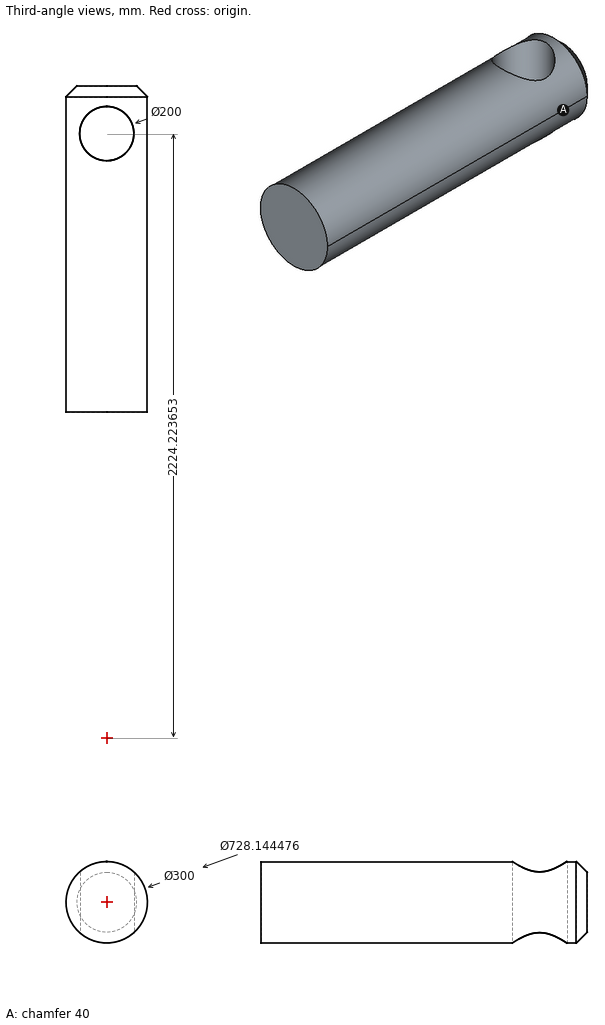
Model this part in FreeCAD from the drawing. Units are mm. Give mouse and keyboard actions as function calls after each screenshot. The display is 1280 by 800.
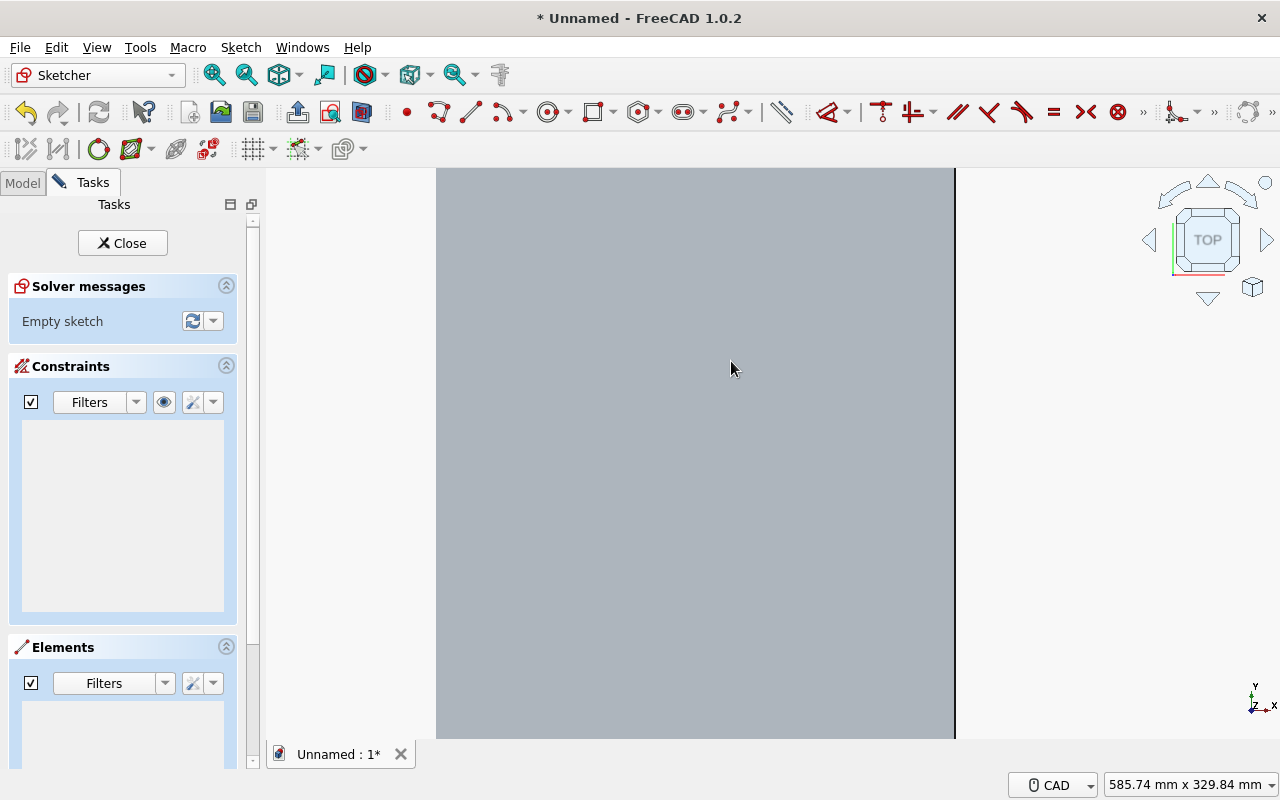
key(g)
key(c)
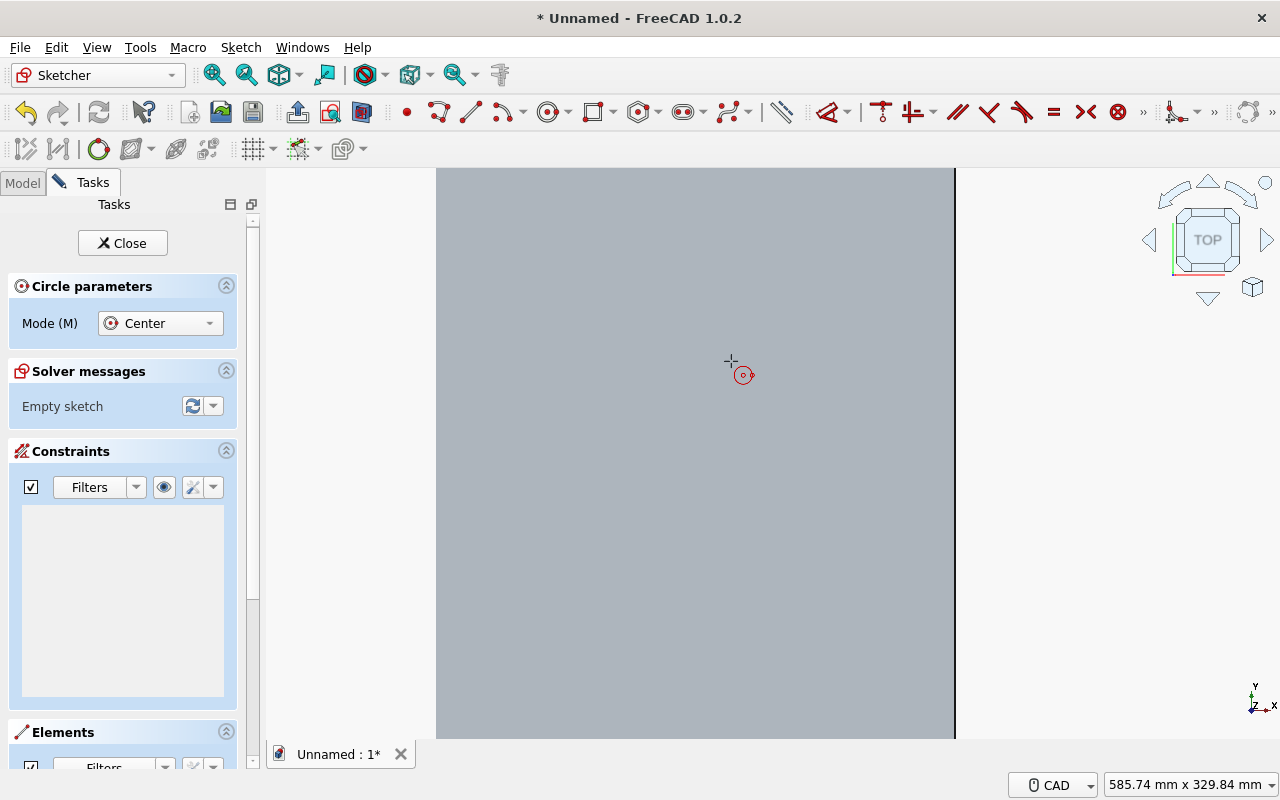
click(695, 452)
move(818, 330)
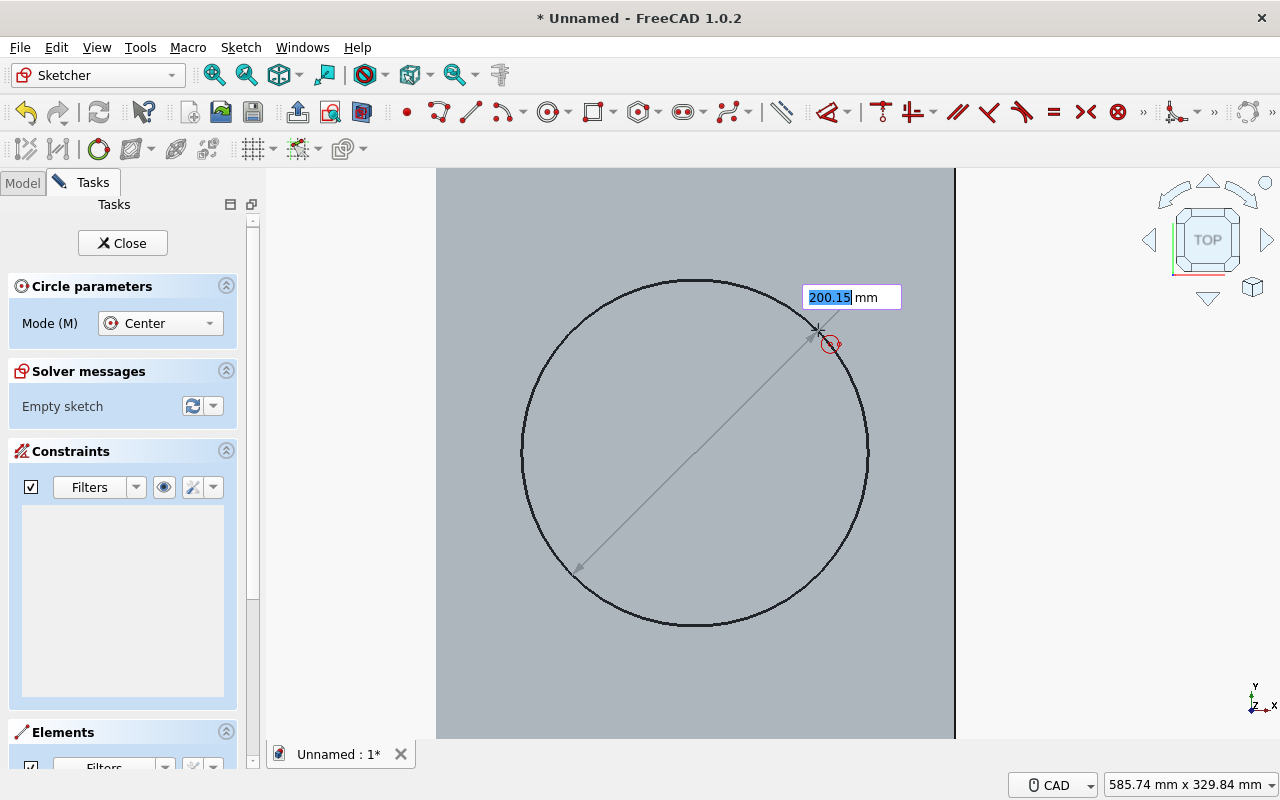
text(200)
key(Return)
key(Escape)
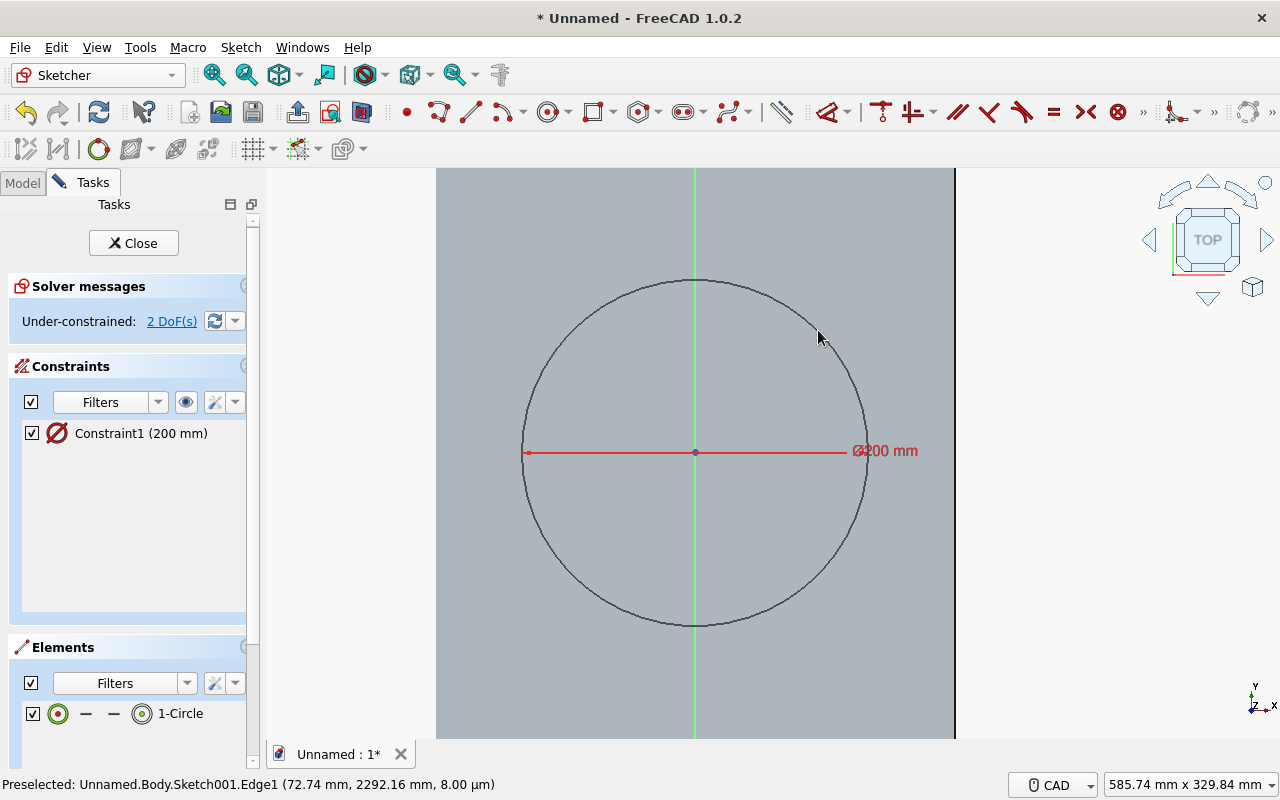
click(695, 453)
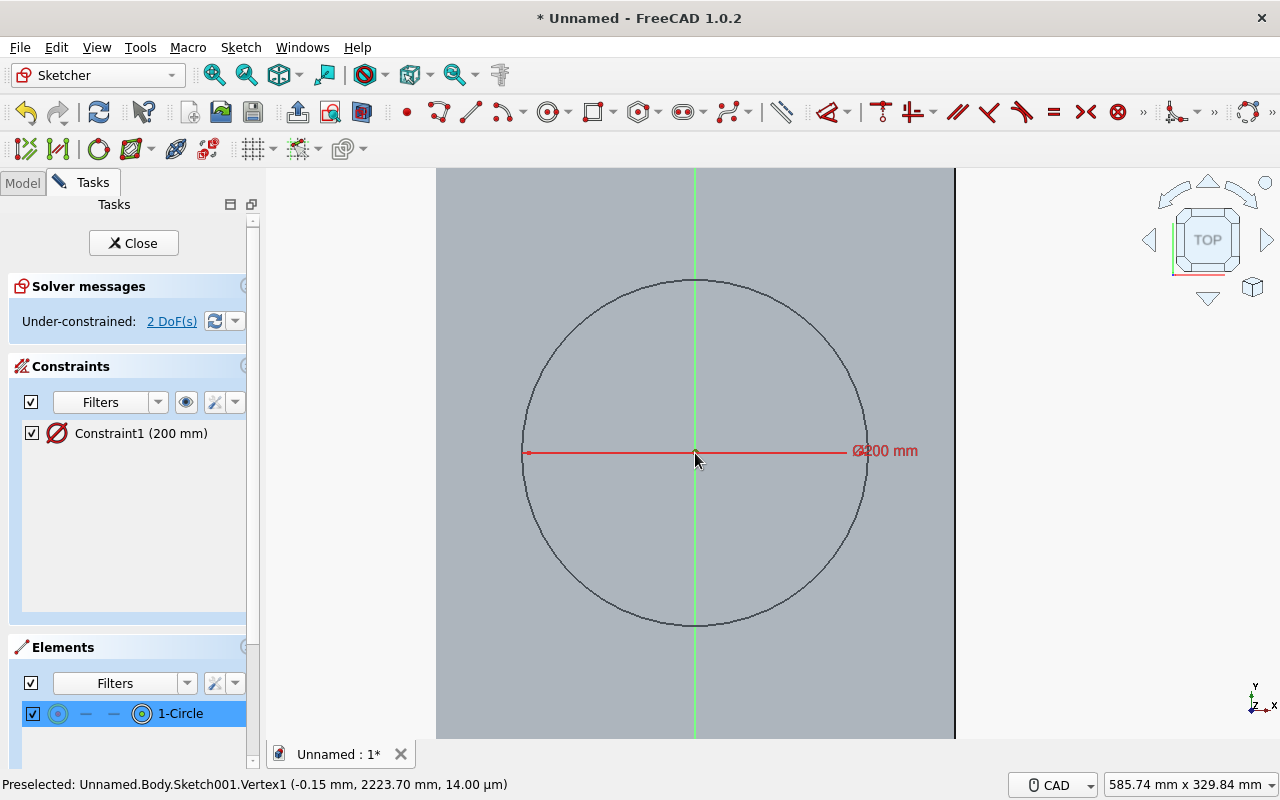
click(695, 674)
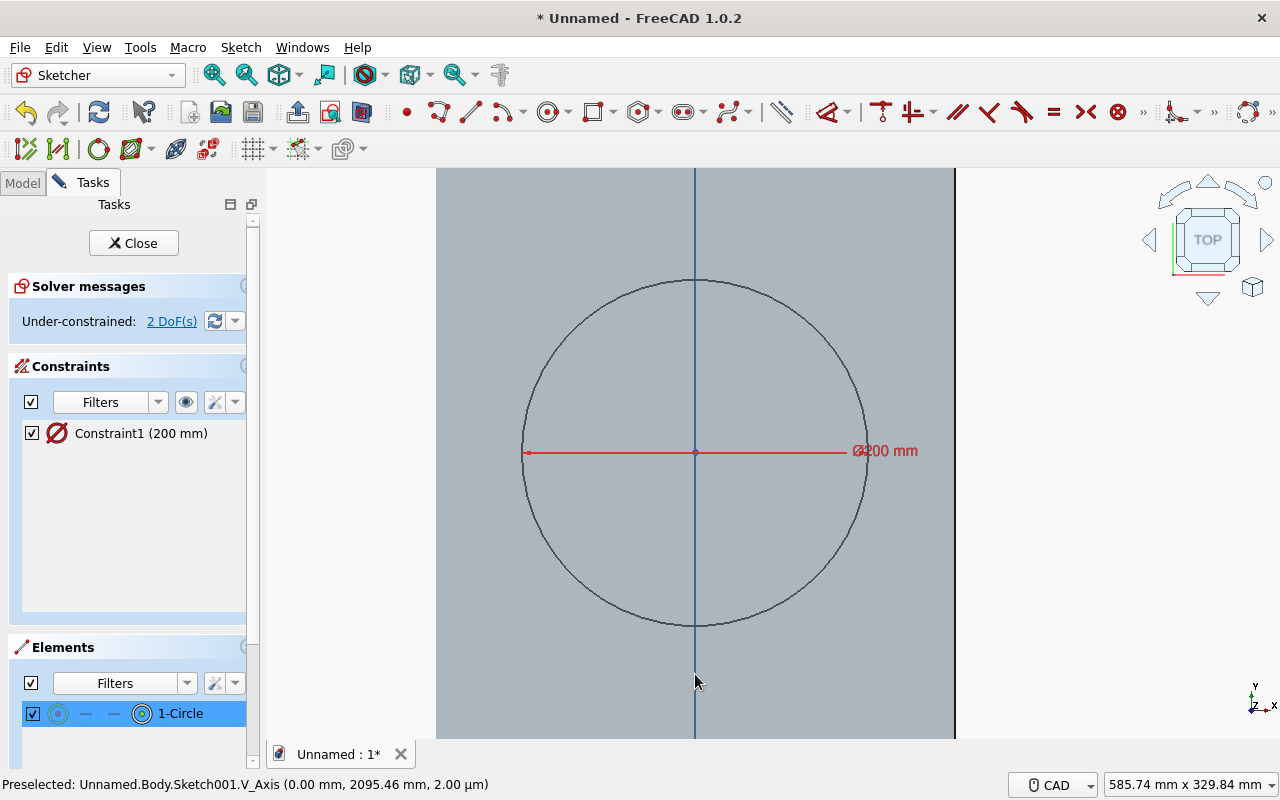
click(882, 112)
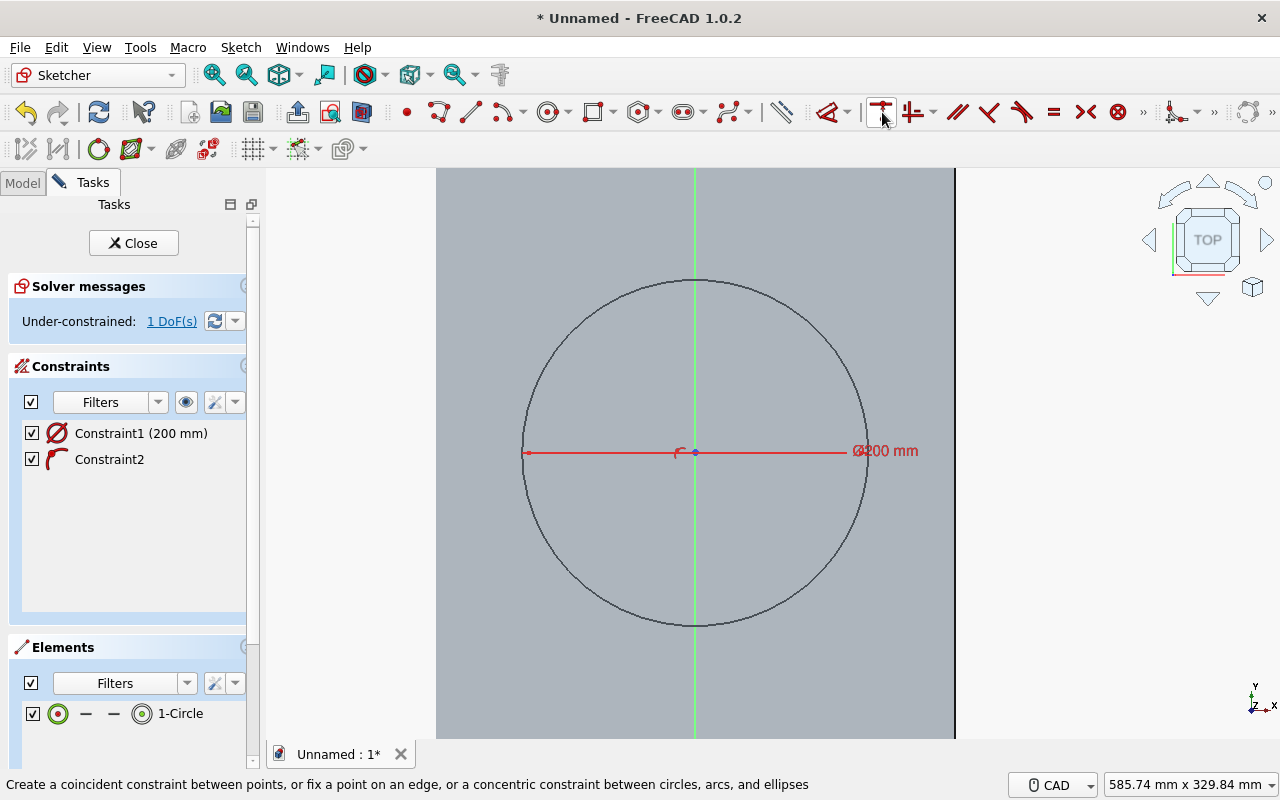
click(695, 453)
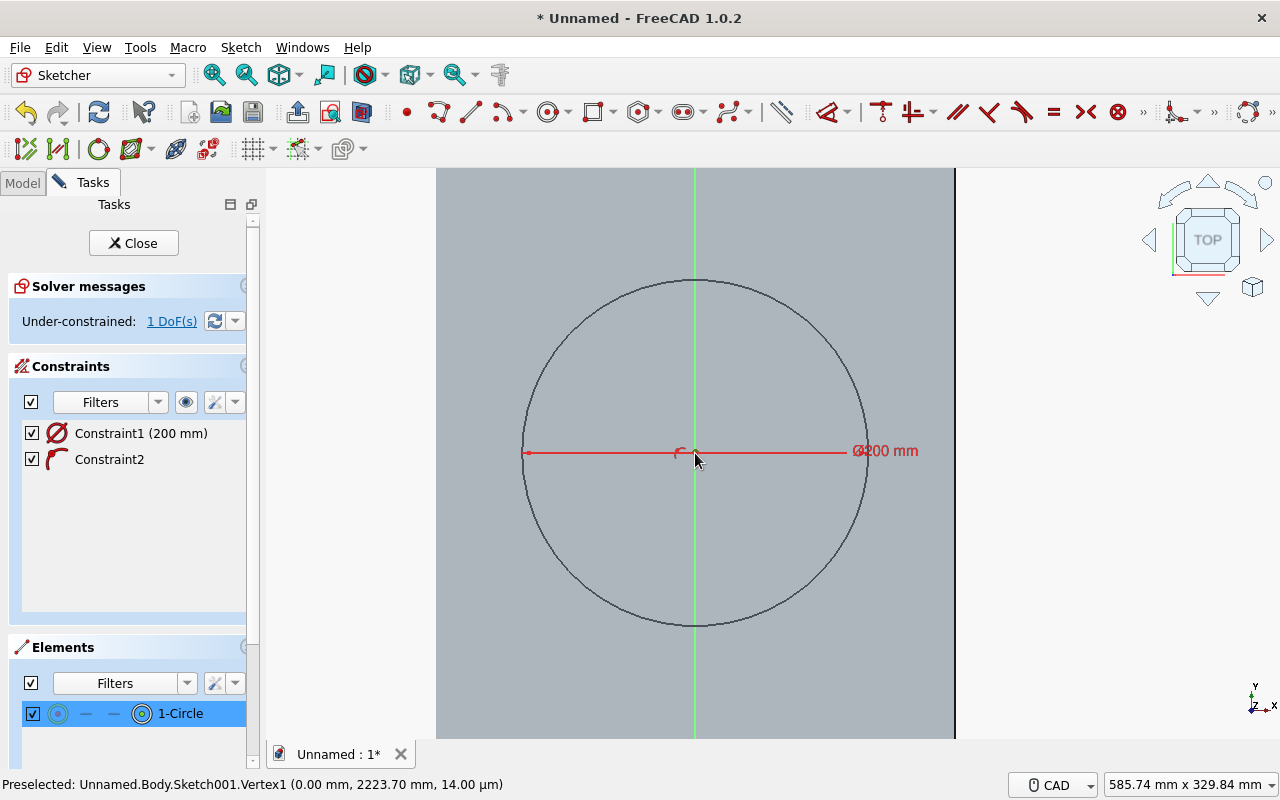
key(i)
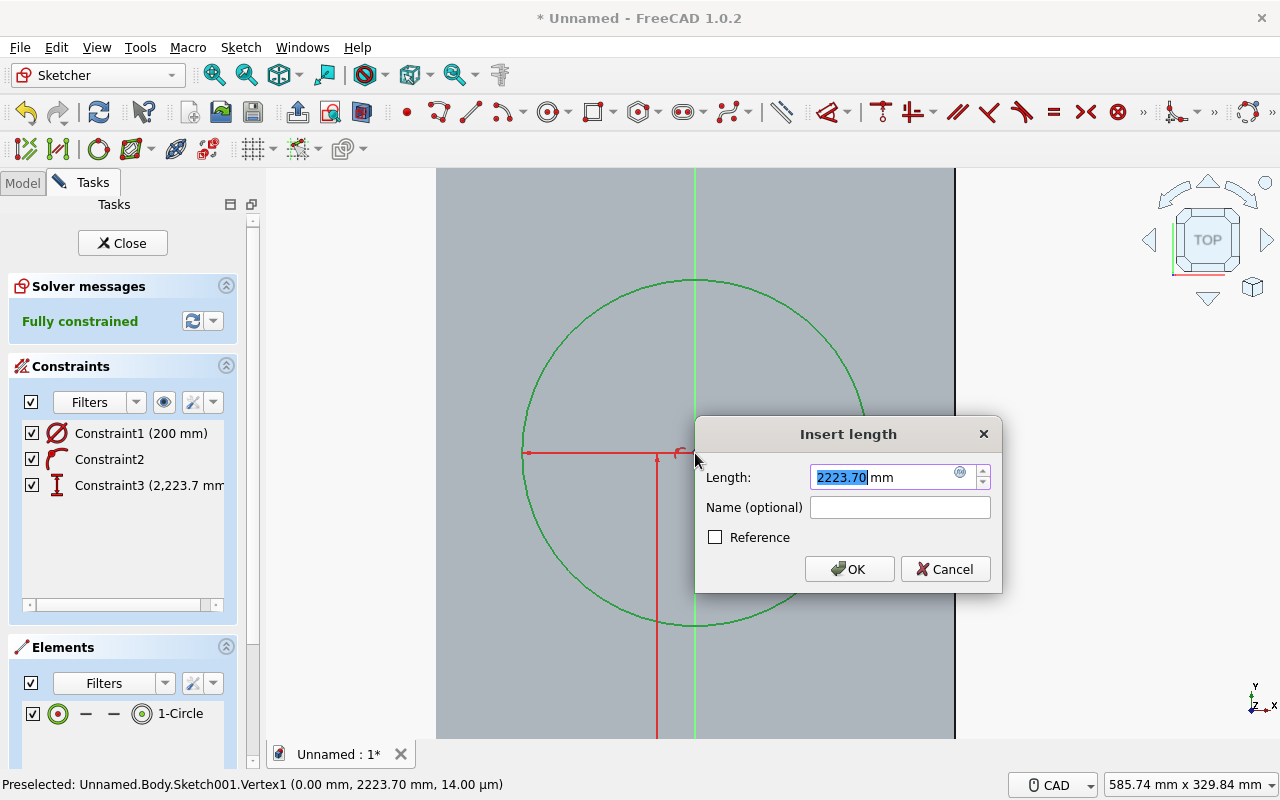
text(2224.223653)
key(Return)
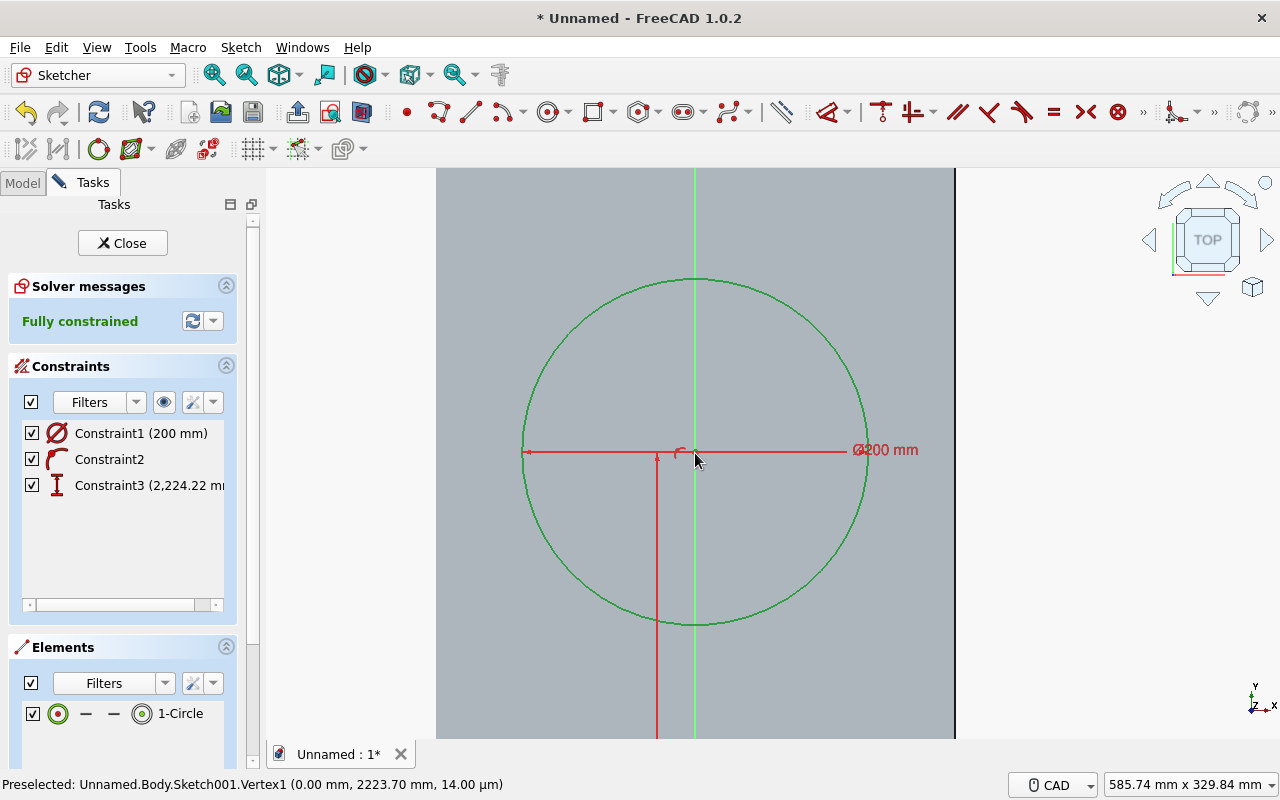
click(123, 243)